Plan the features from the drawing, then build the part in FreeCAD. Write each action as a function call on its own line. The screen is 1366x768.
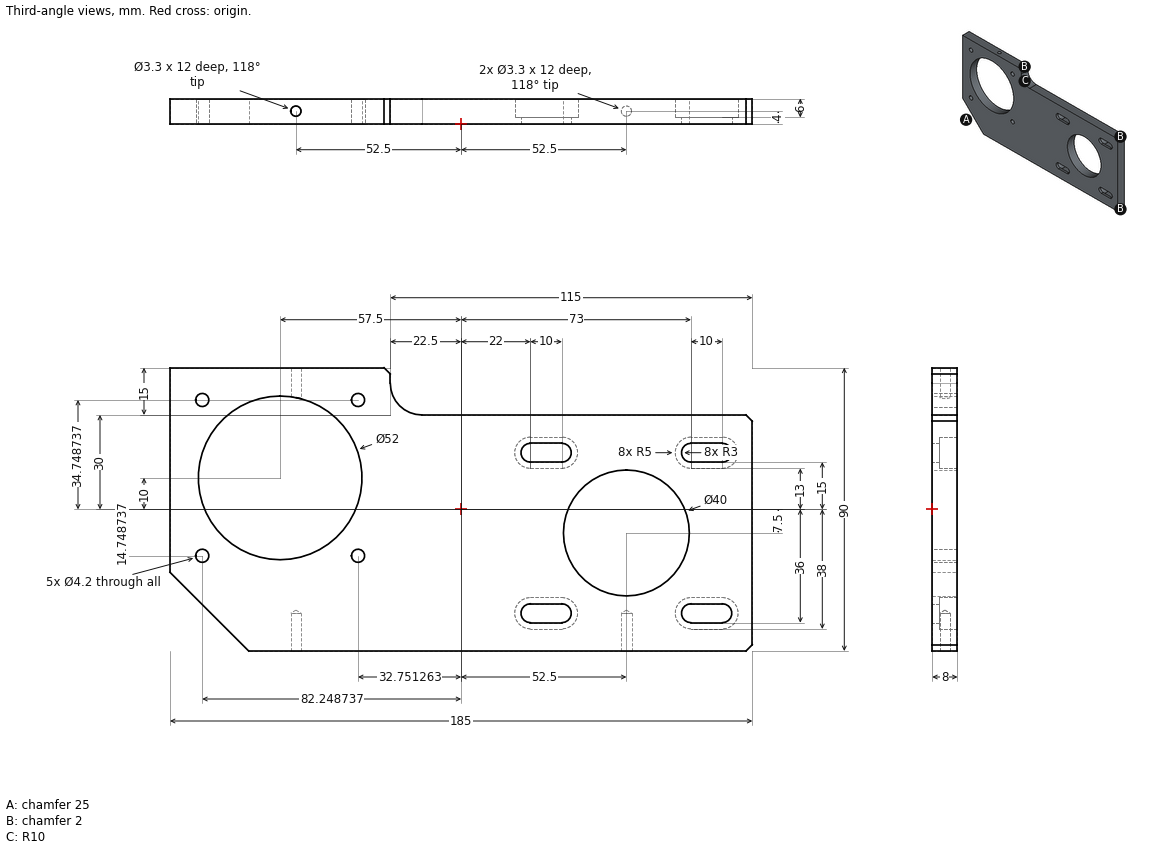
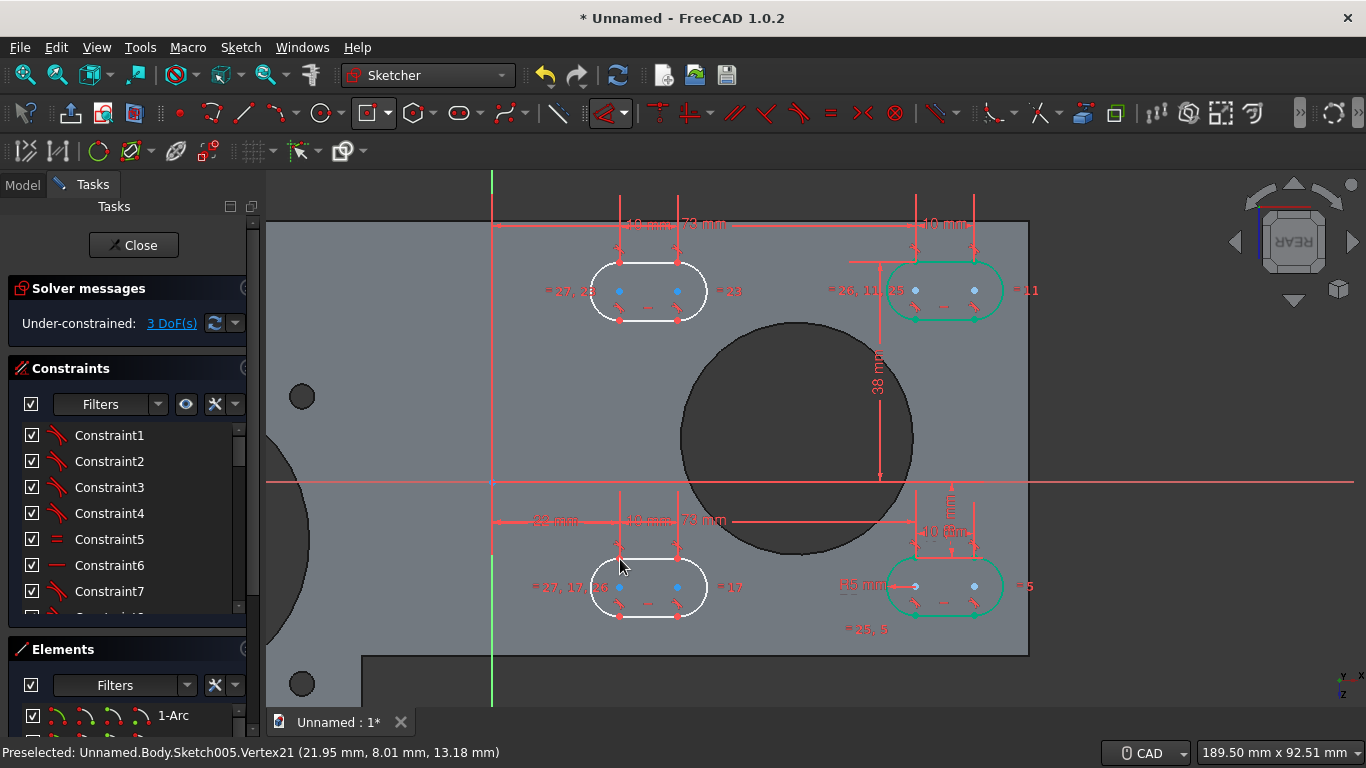
click(620, 559)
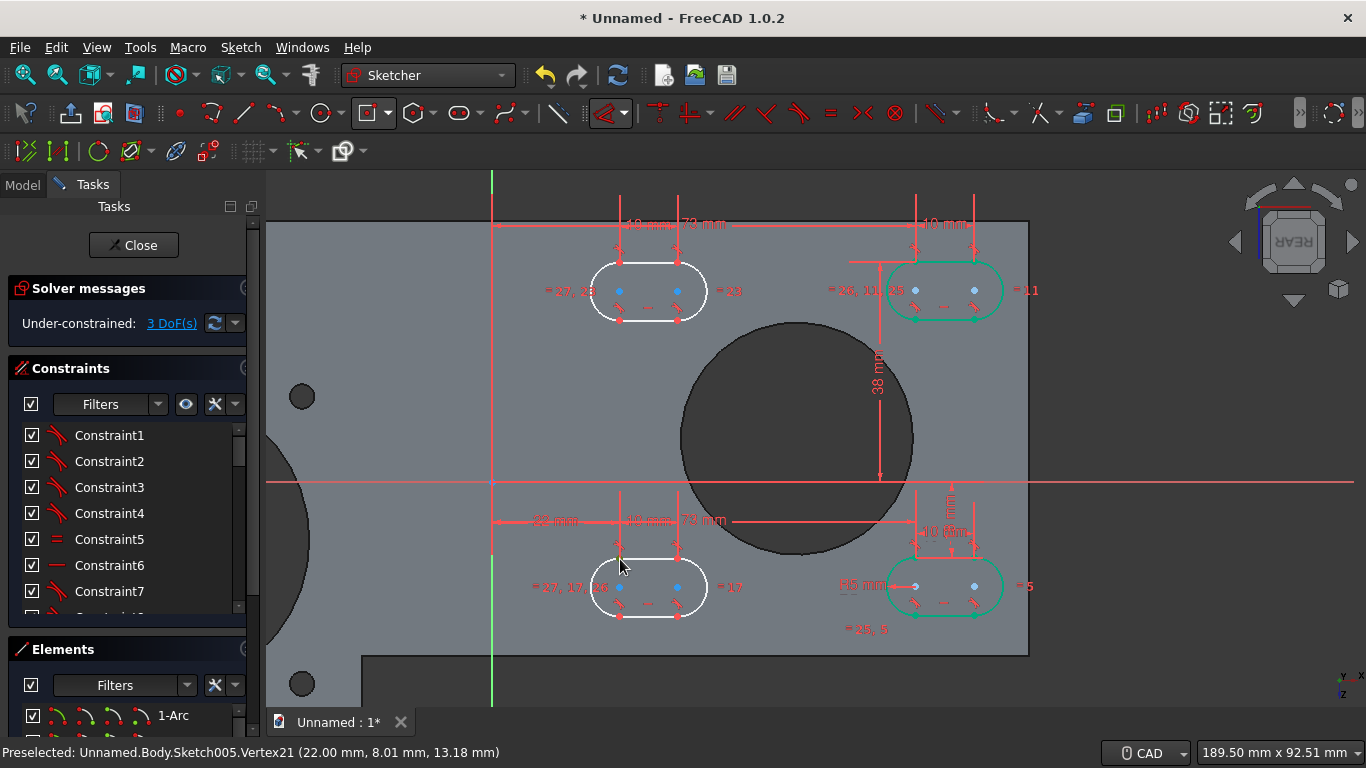
click(626, 114)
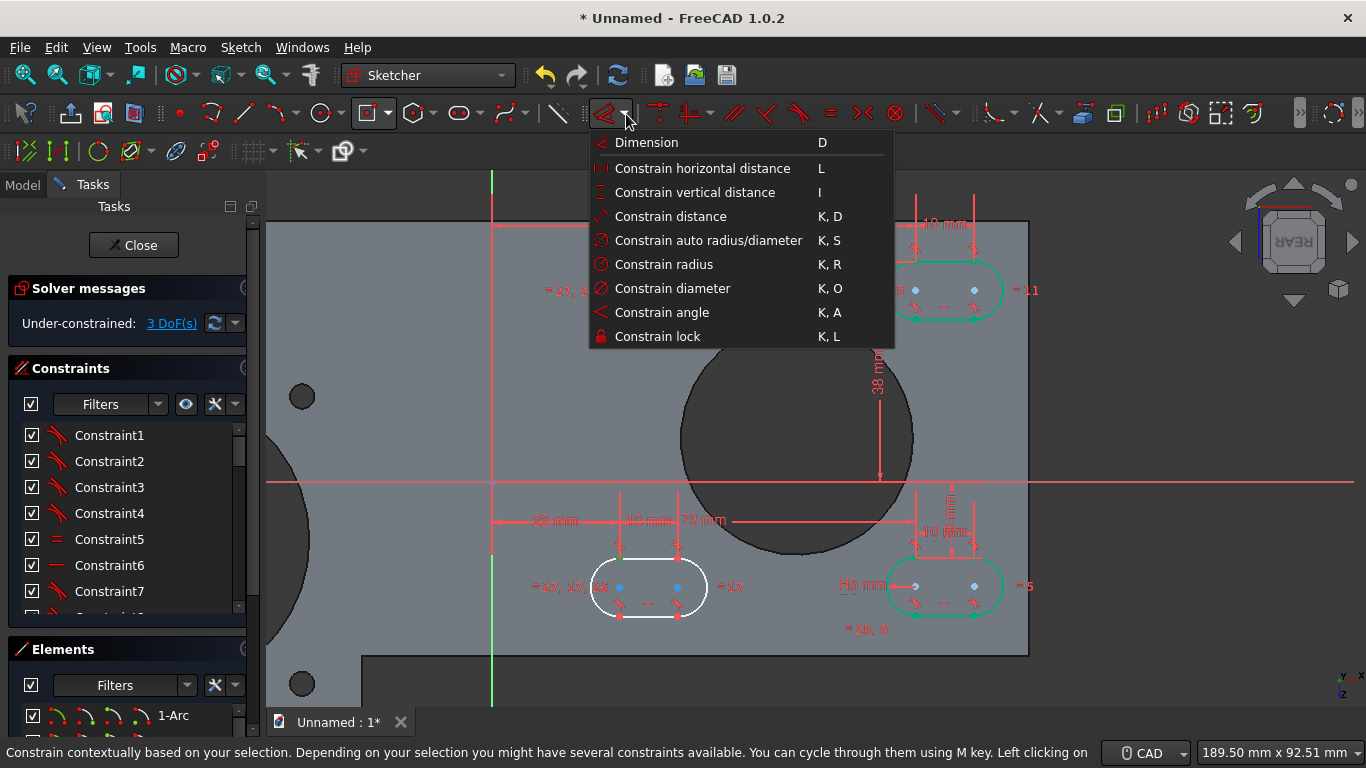
click(742, 192)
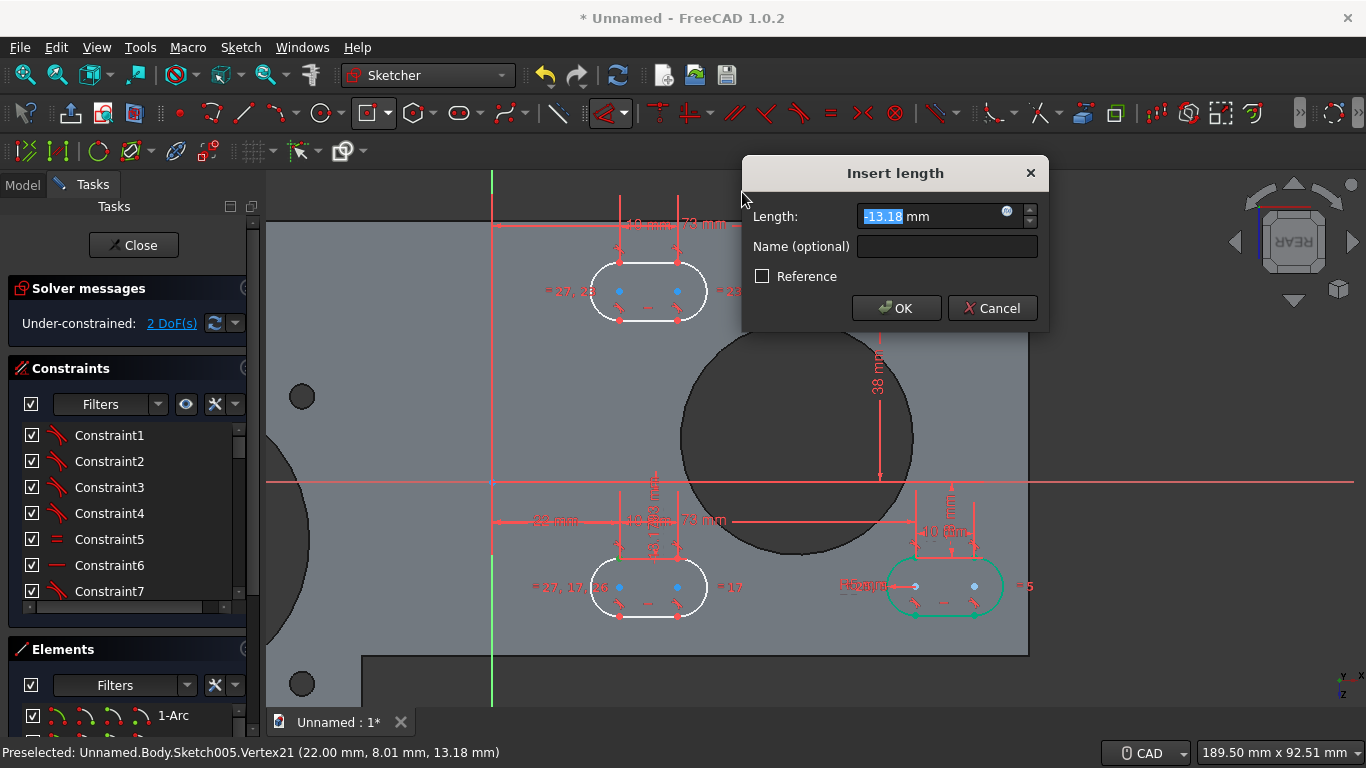
text(-13)
key(Return)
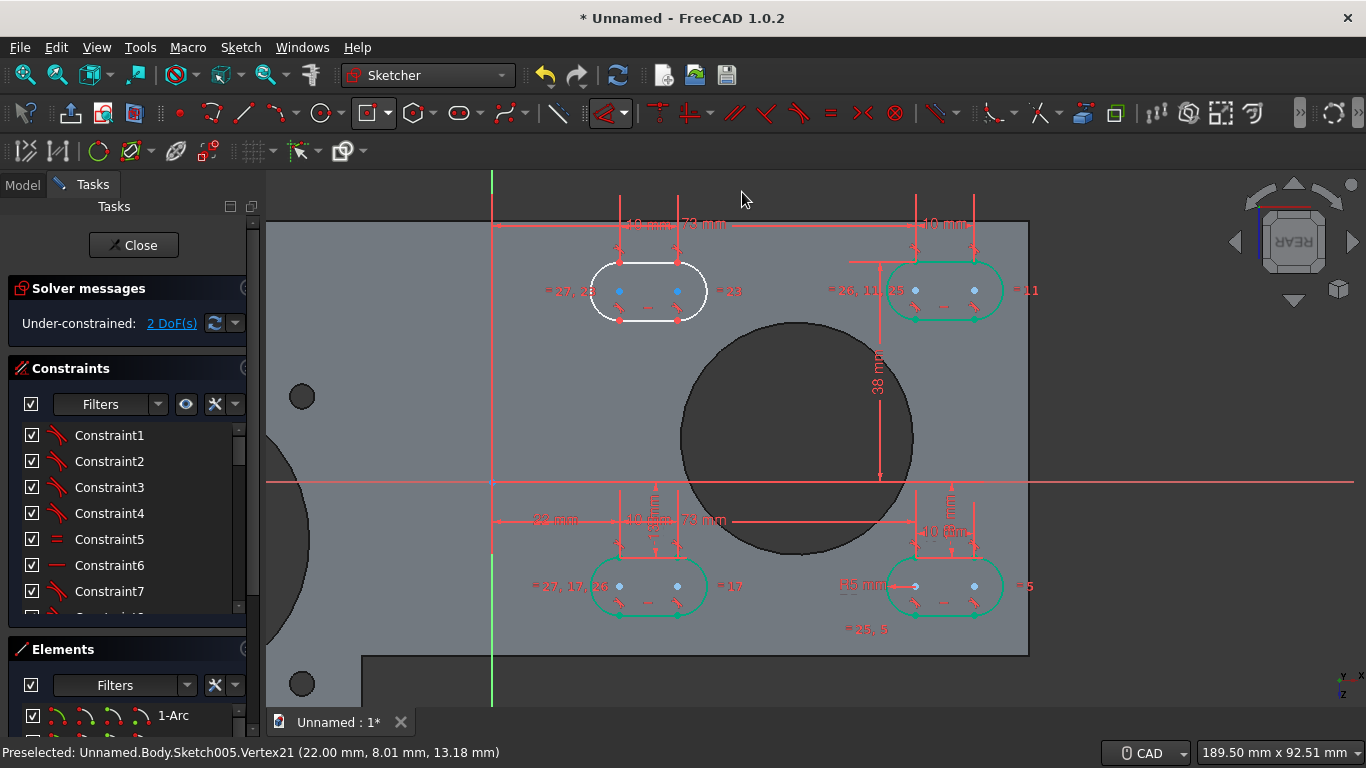
click(620, 263)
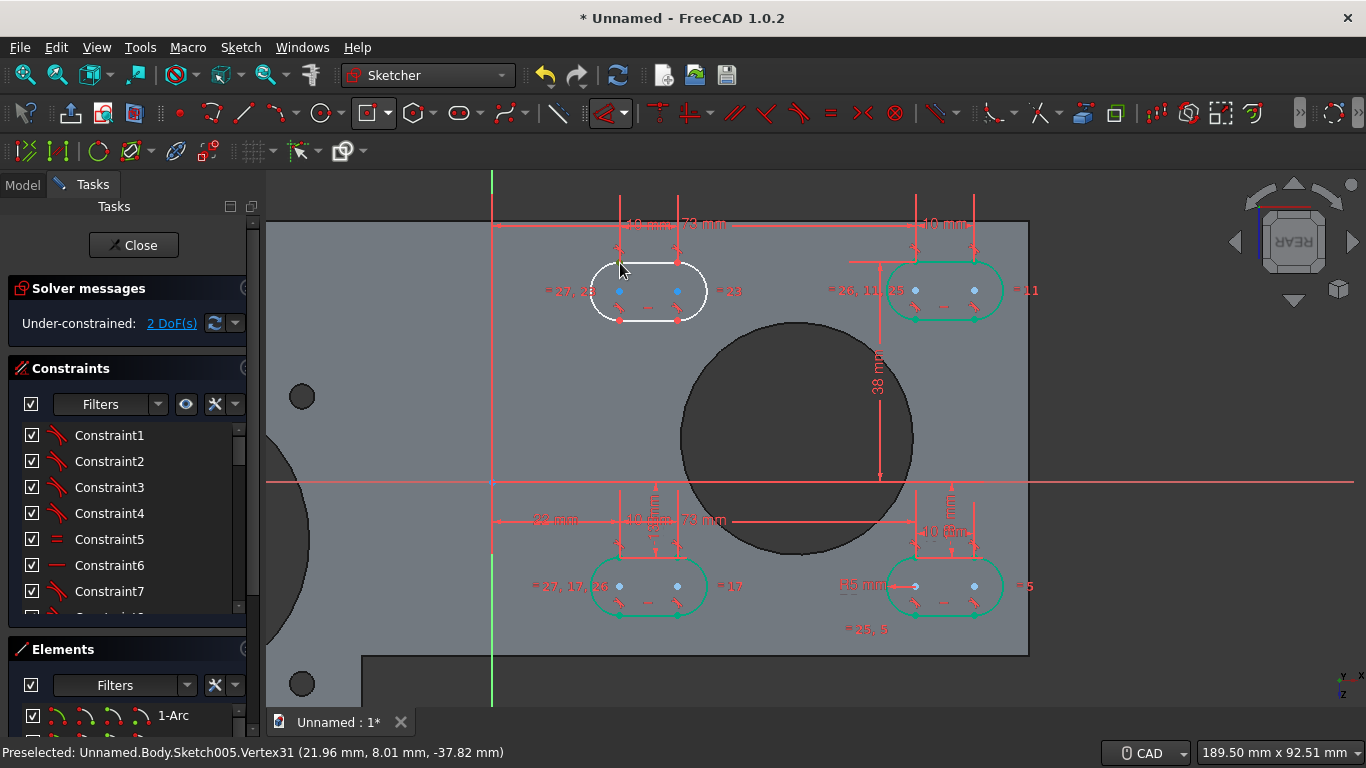
key(l)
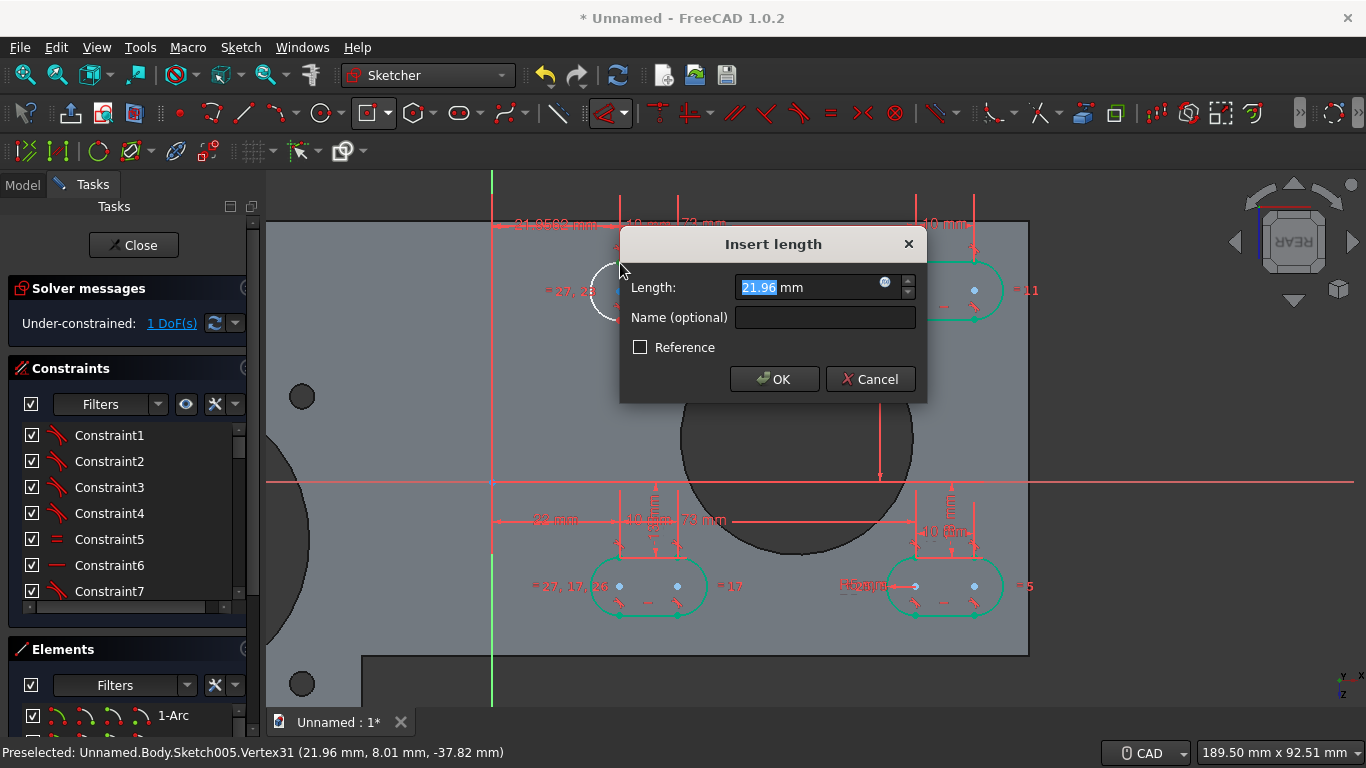
text(22)
key(Return)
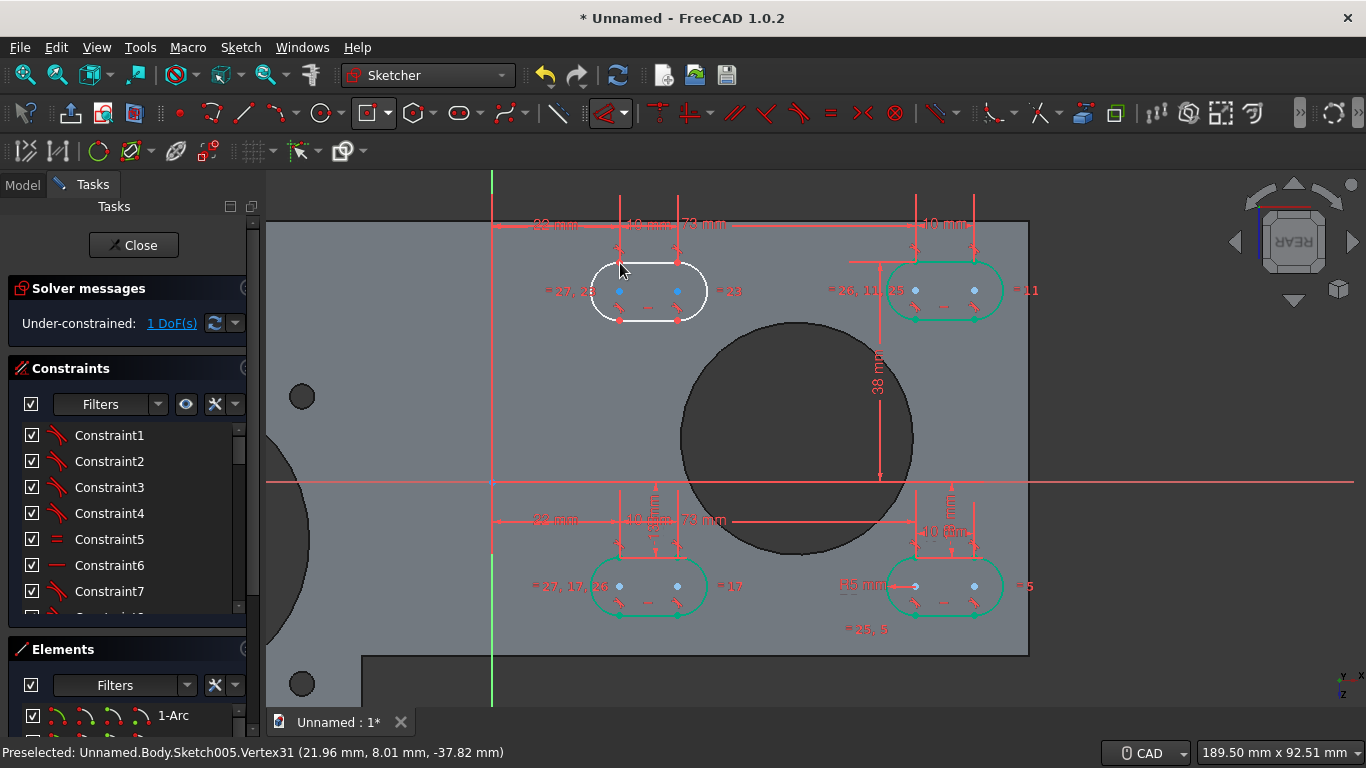
click(620, 263)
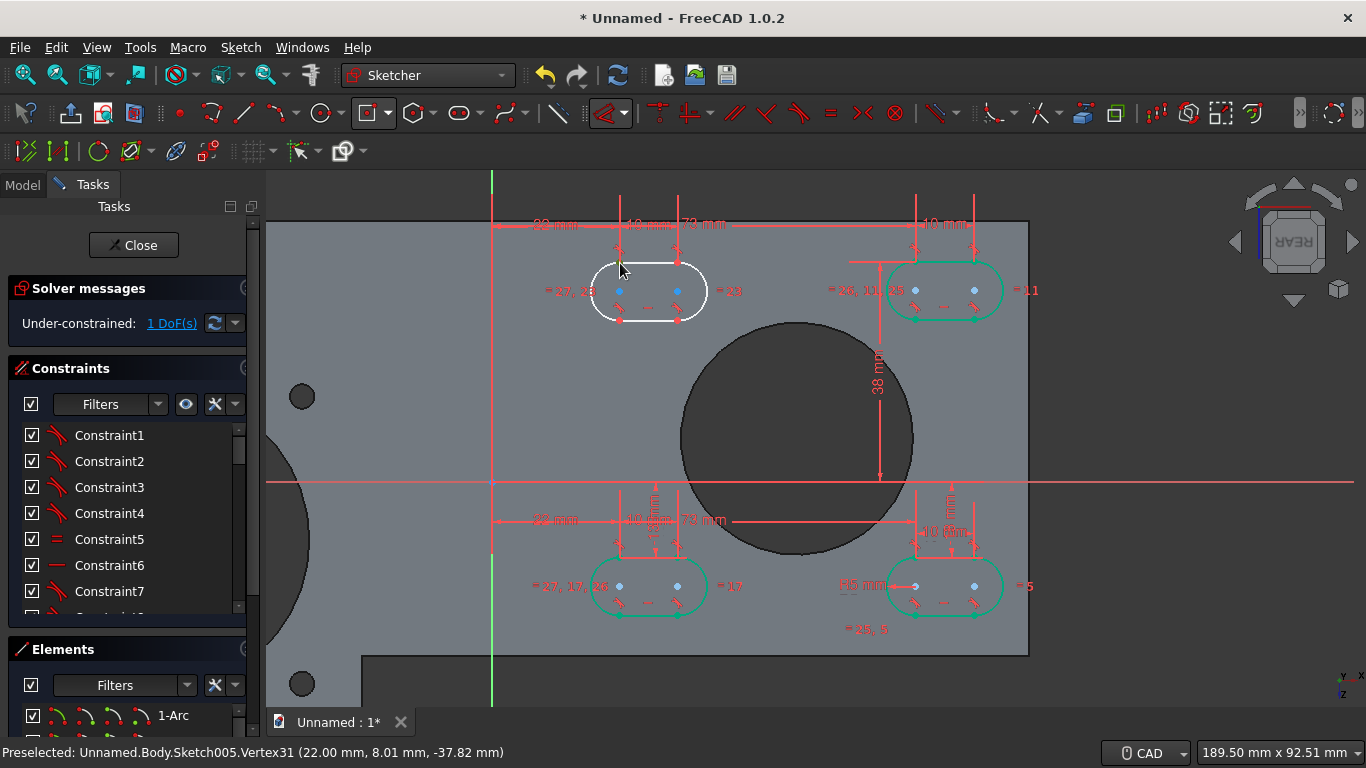
key(i)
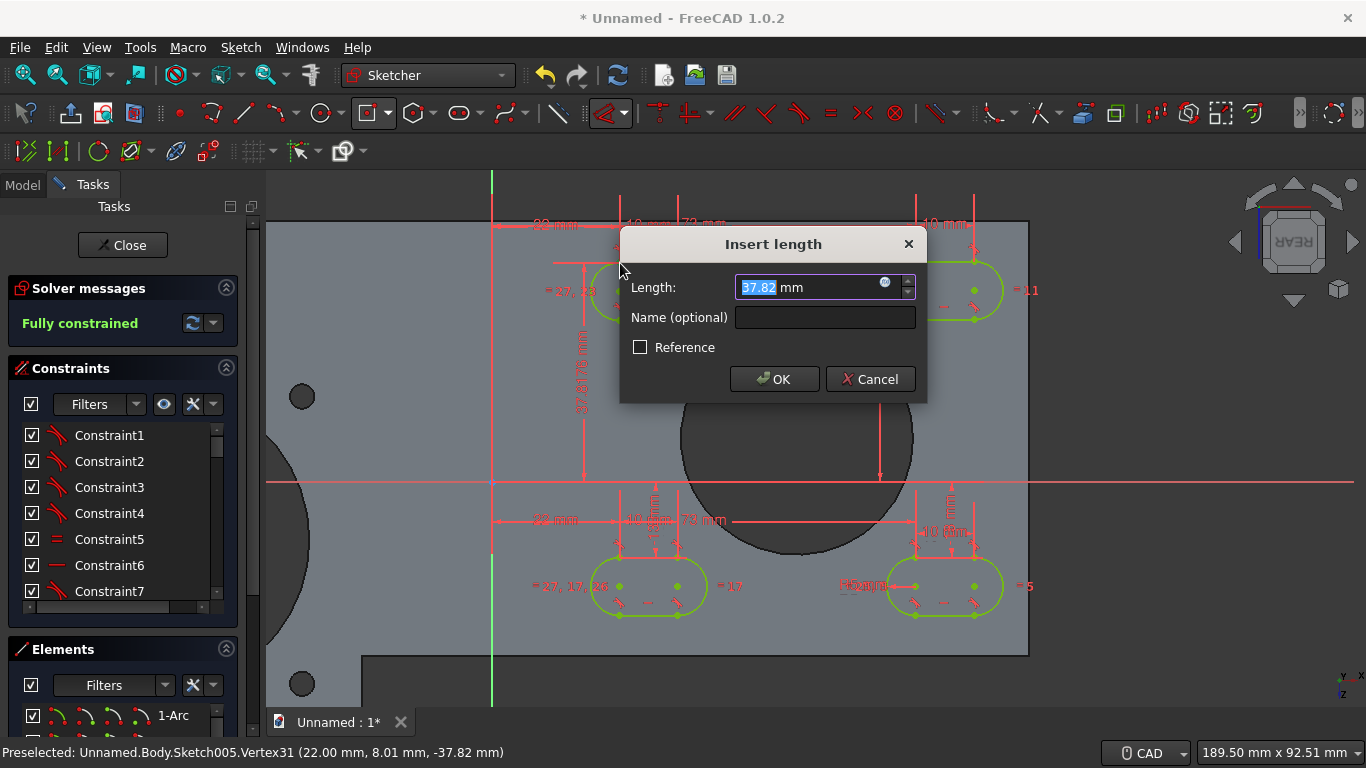
text(38)
key(Return)